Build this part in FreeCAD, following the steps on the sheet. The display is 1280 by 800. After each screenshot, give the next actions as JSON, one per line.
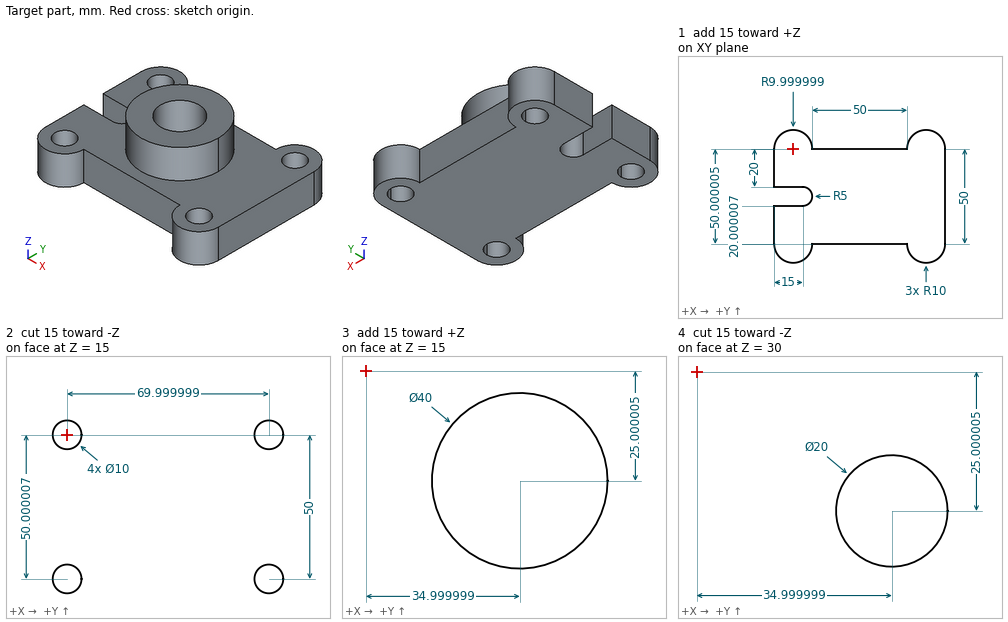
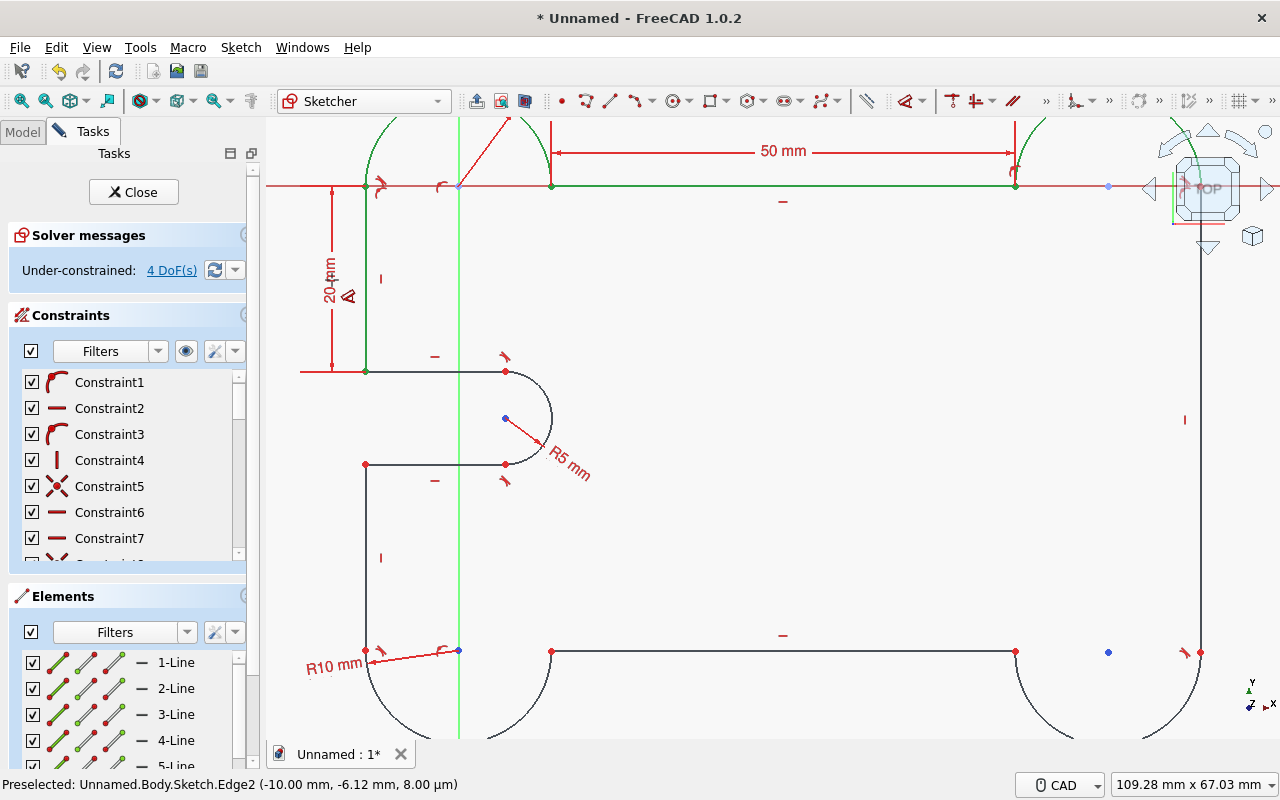
{"action": "left_click", "coordinate": [408, 465]}
{"action": "left_click", "coordinate": [436, 499]}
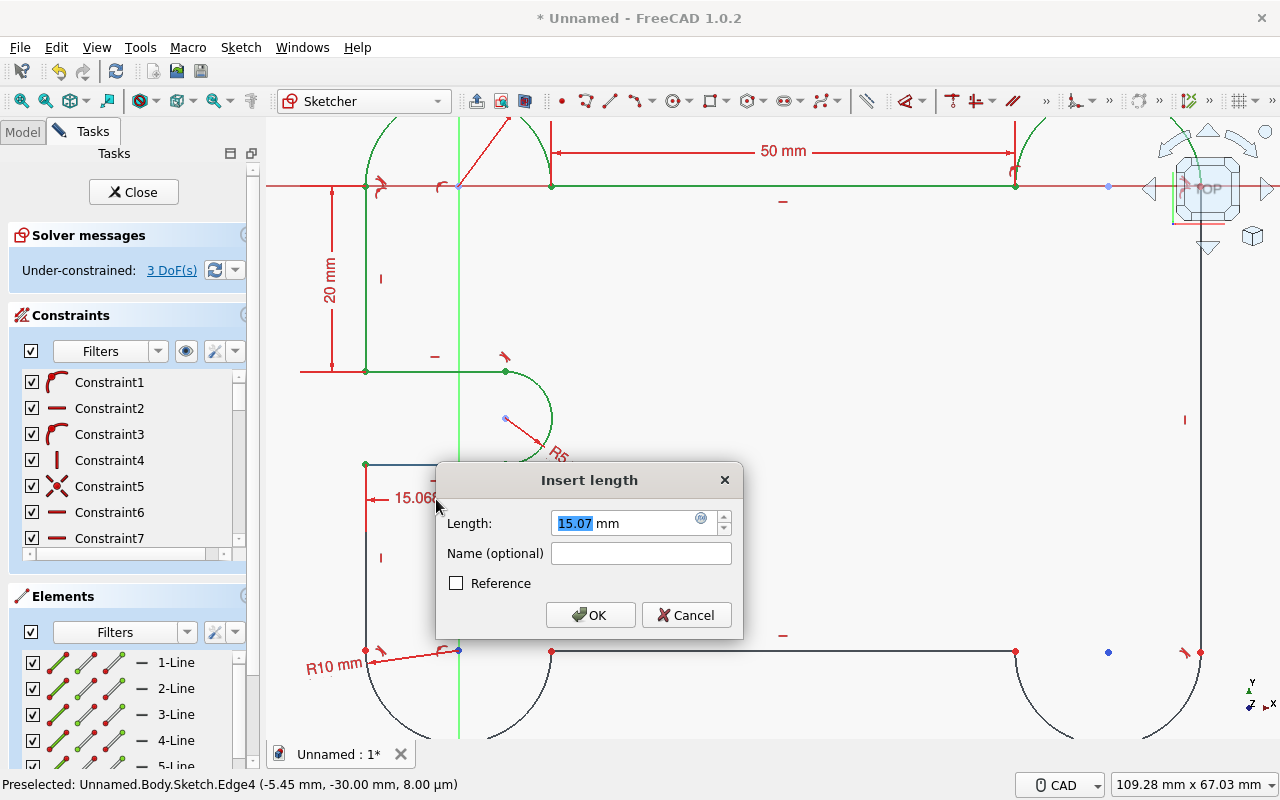
{"action": "type", "text": "15"}
{"action": "key", "text": "Return"}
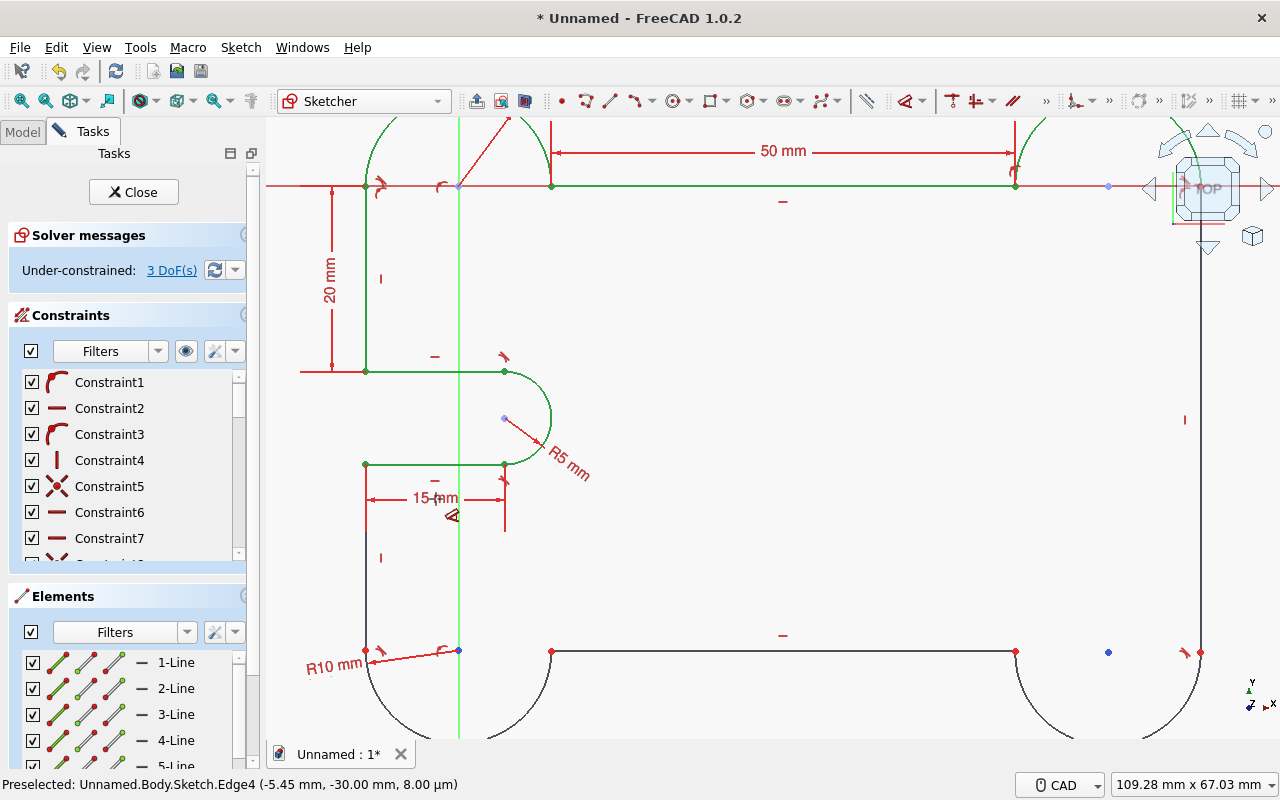
{"action": "scroll", "coordinate": [544, 448], "scroll_direction": "down", "scroll_amount": 2}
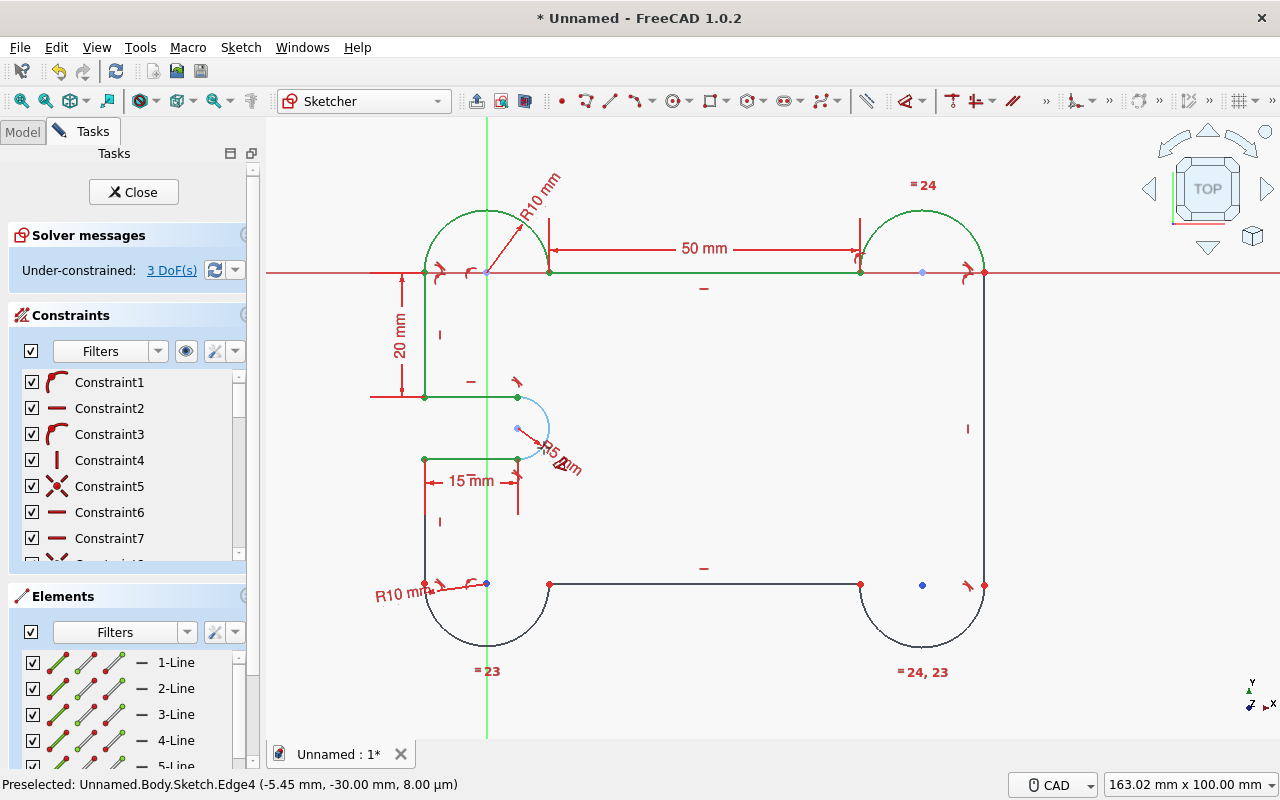
{"action": "left_click", "coordinate": [984, 492]}
{"action": "left_click", "coordinate": [1018, 429]}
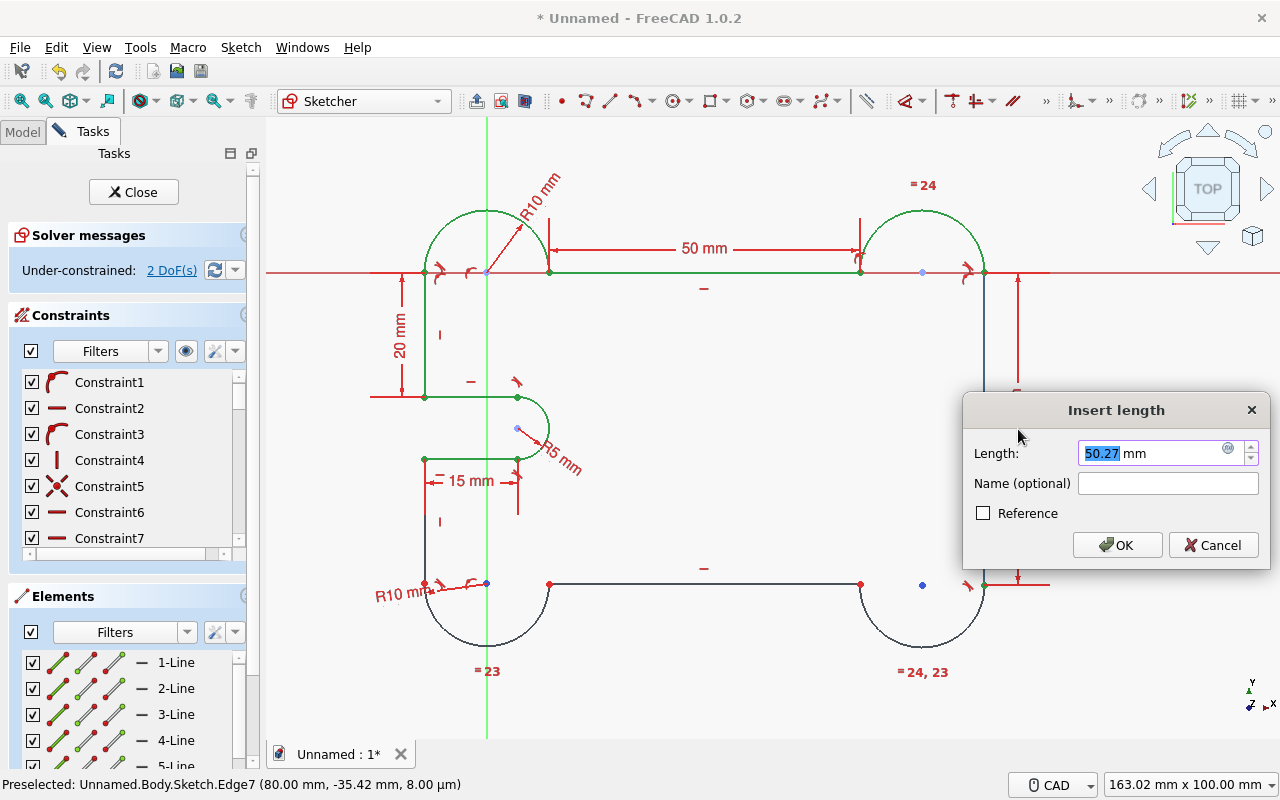
{"action": "type", "text": "50"}
{"action": "key", "text": "Return"}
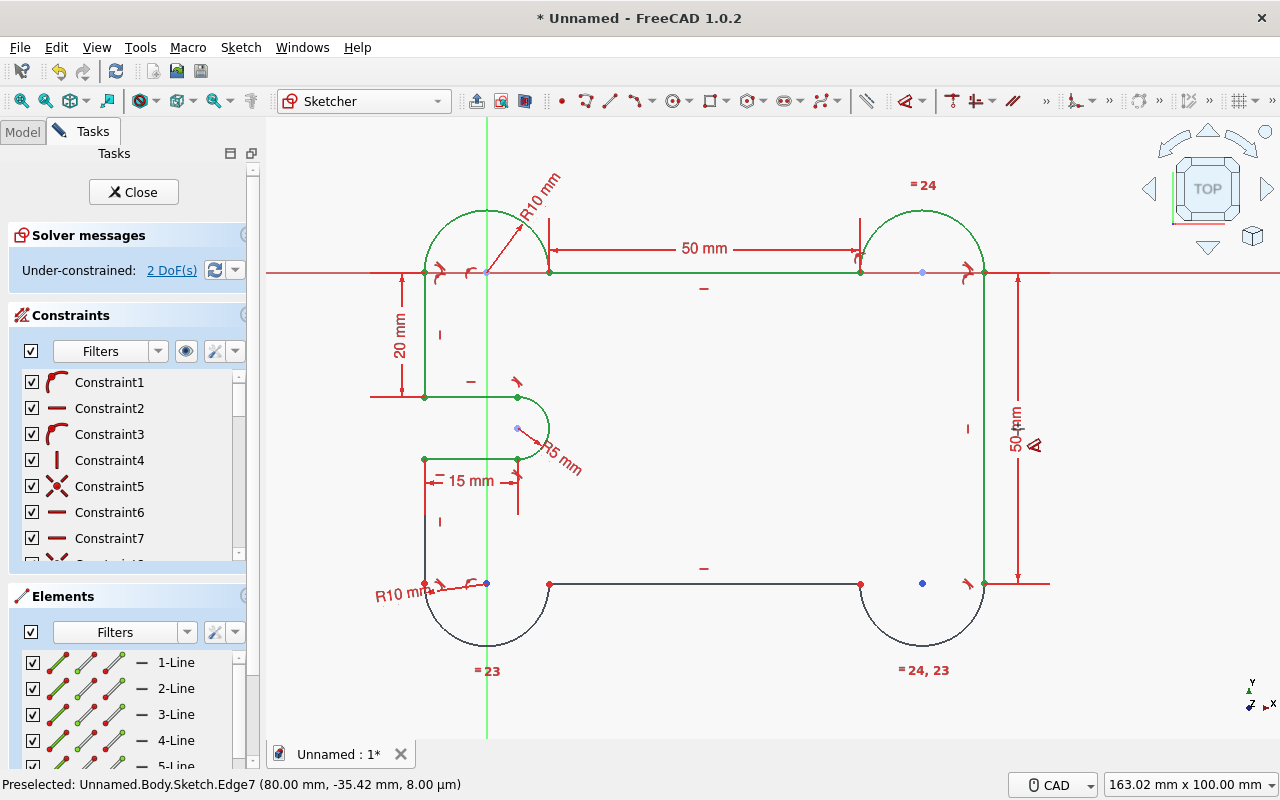
{"action": "left_click", "coordinate": [425, 497]}
{"action": "left_click", "coordinate": [391, 522]}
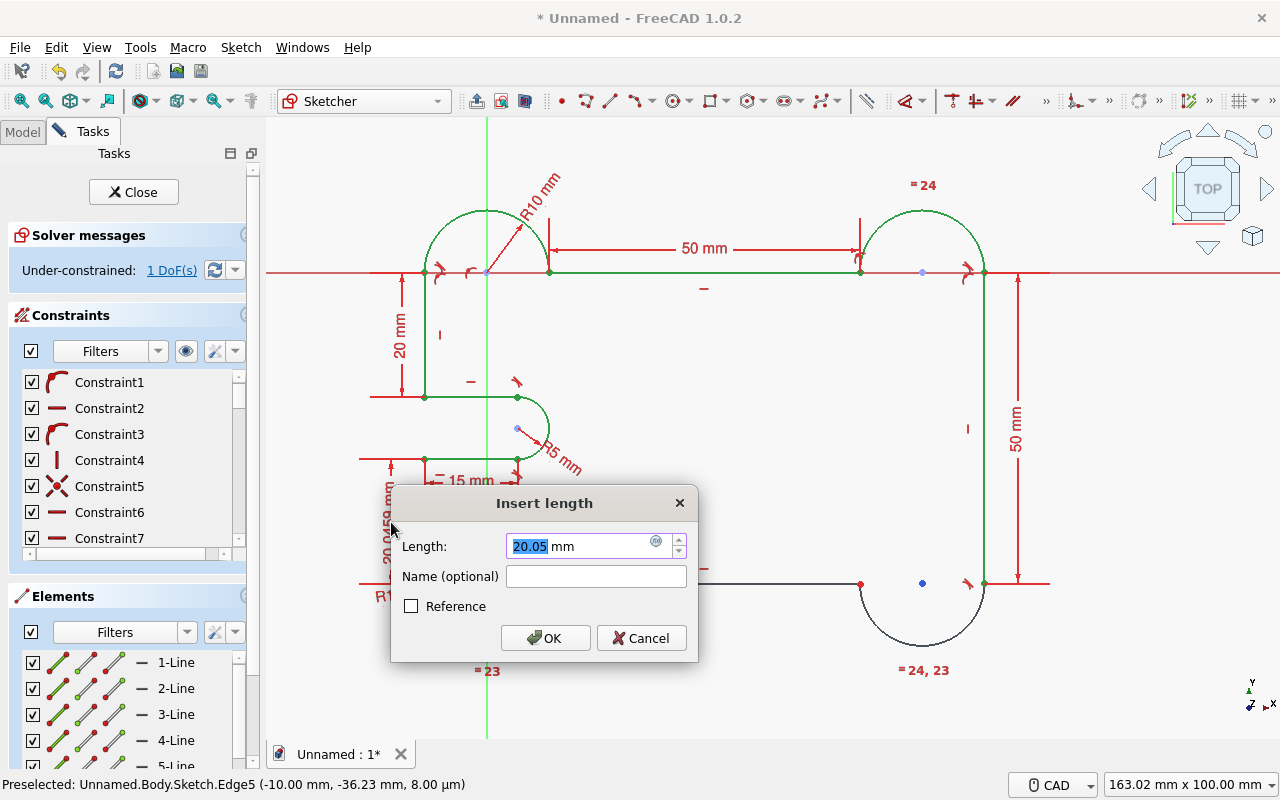
{"action": "type", "text": "20.000007"}
{"action": "key", "text": "Return"}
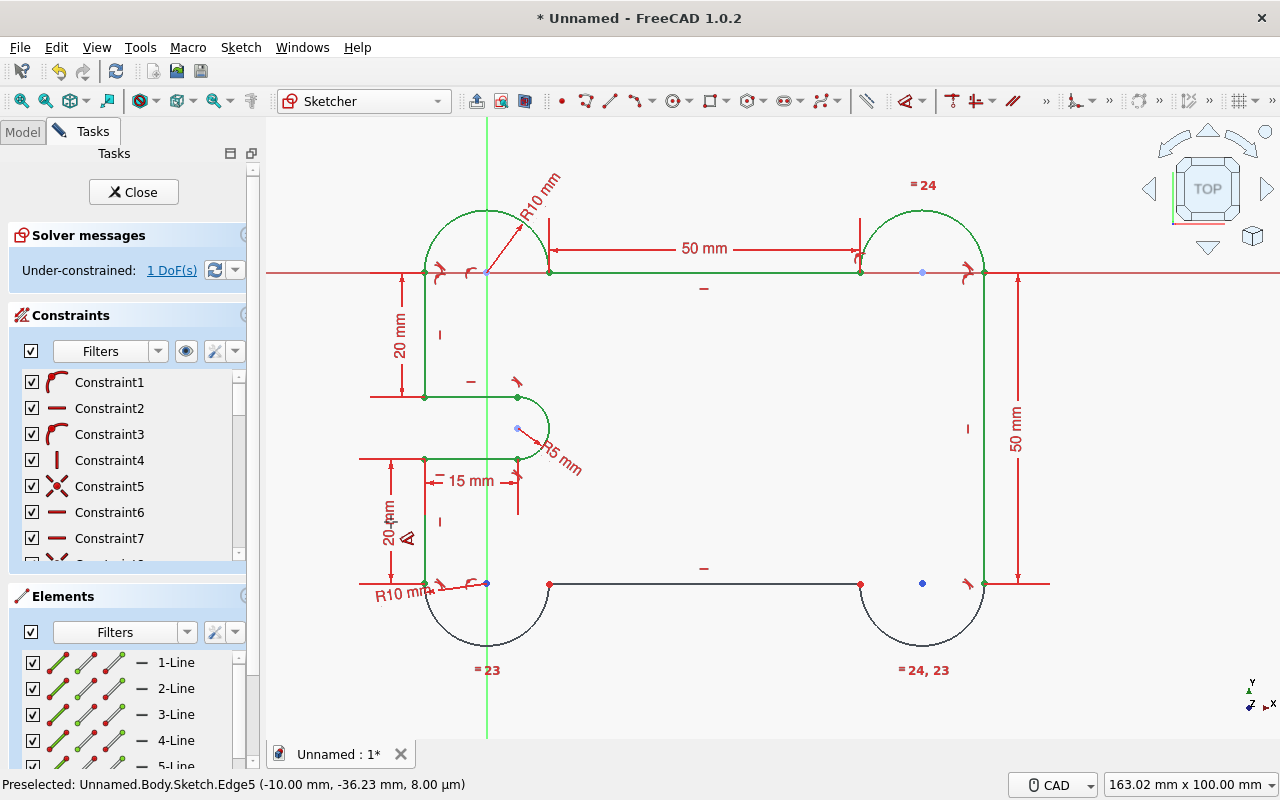
{"action": "left_click", "coordinate": [549, 584]}
{"action": "left_click", "coordinate": [453, 428]}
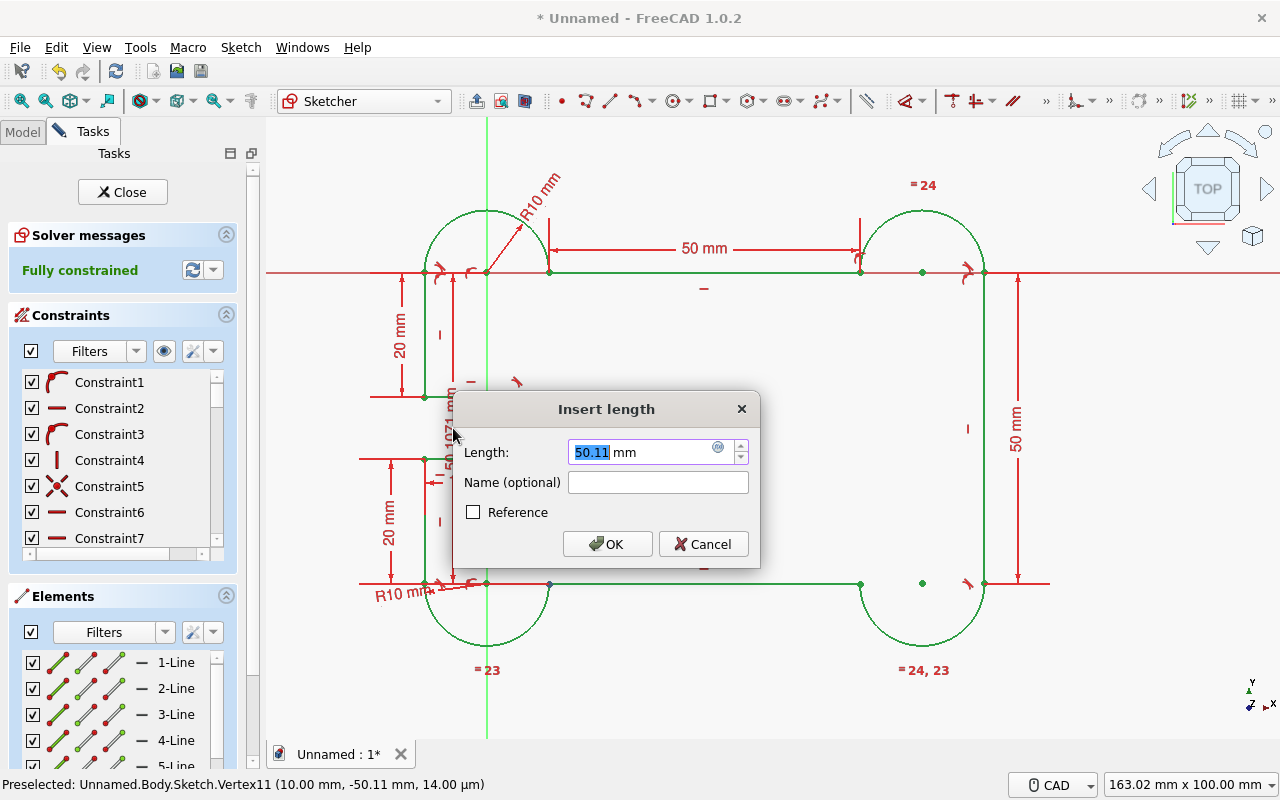
{"action": "type", "text": "50.000005"}
{"action": "key", "text": "Return"}
{"action": "key", "text": "Escape"}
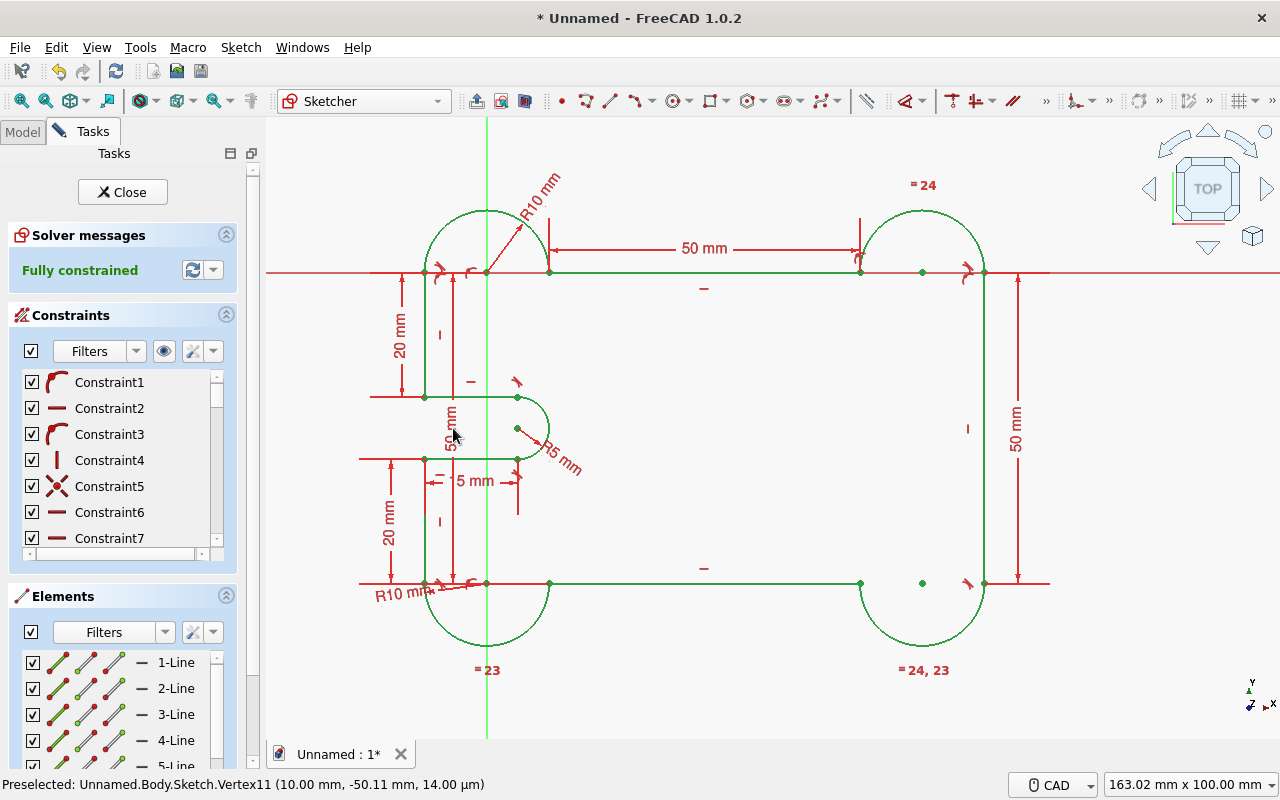
{"action": "left_click", "coordinate": [123, 192]}